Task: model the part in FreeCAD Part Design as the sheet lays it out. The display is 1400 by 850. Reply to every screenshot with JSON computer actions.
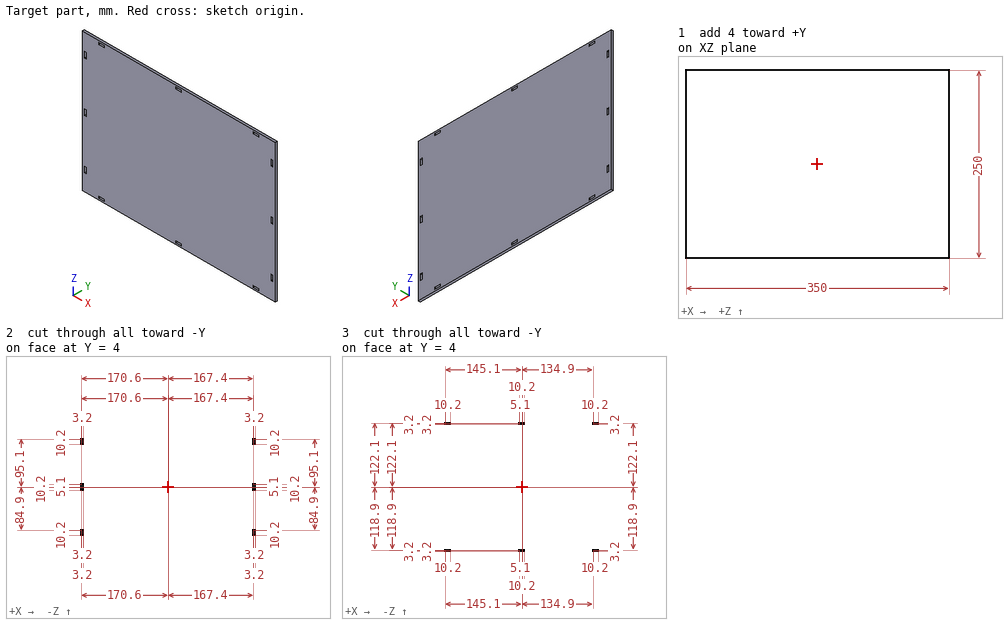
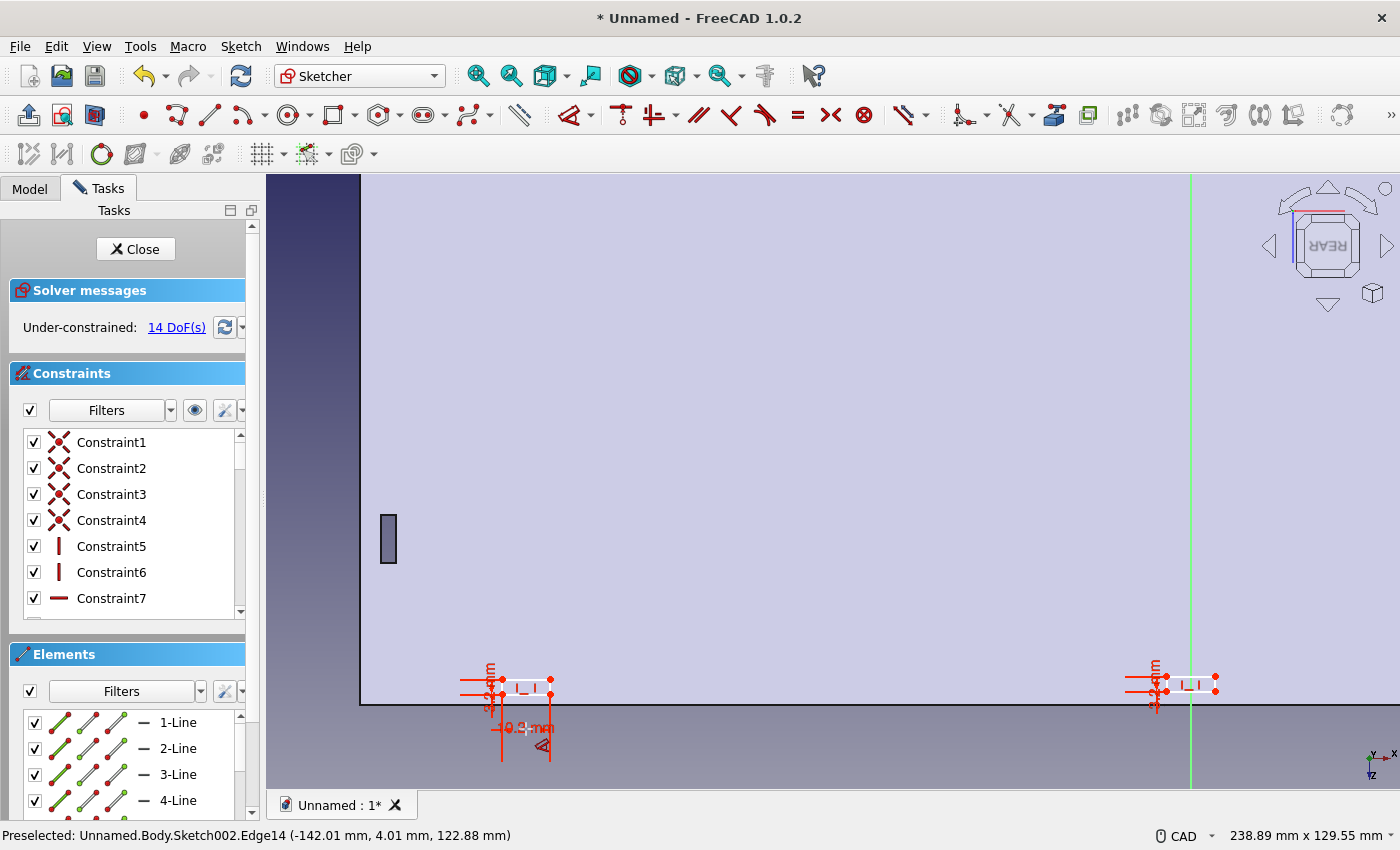
{"action": "scroll", "coordinate": [516, 697], "scroll_direction": "down", "scroll_amount": 5}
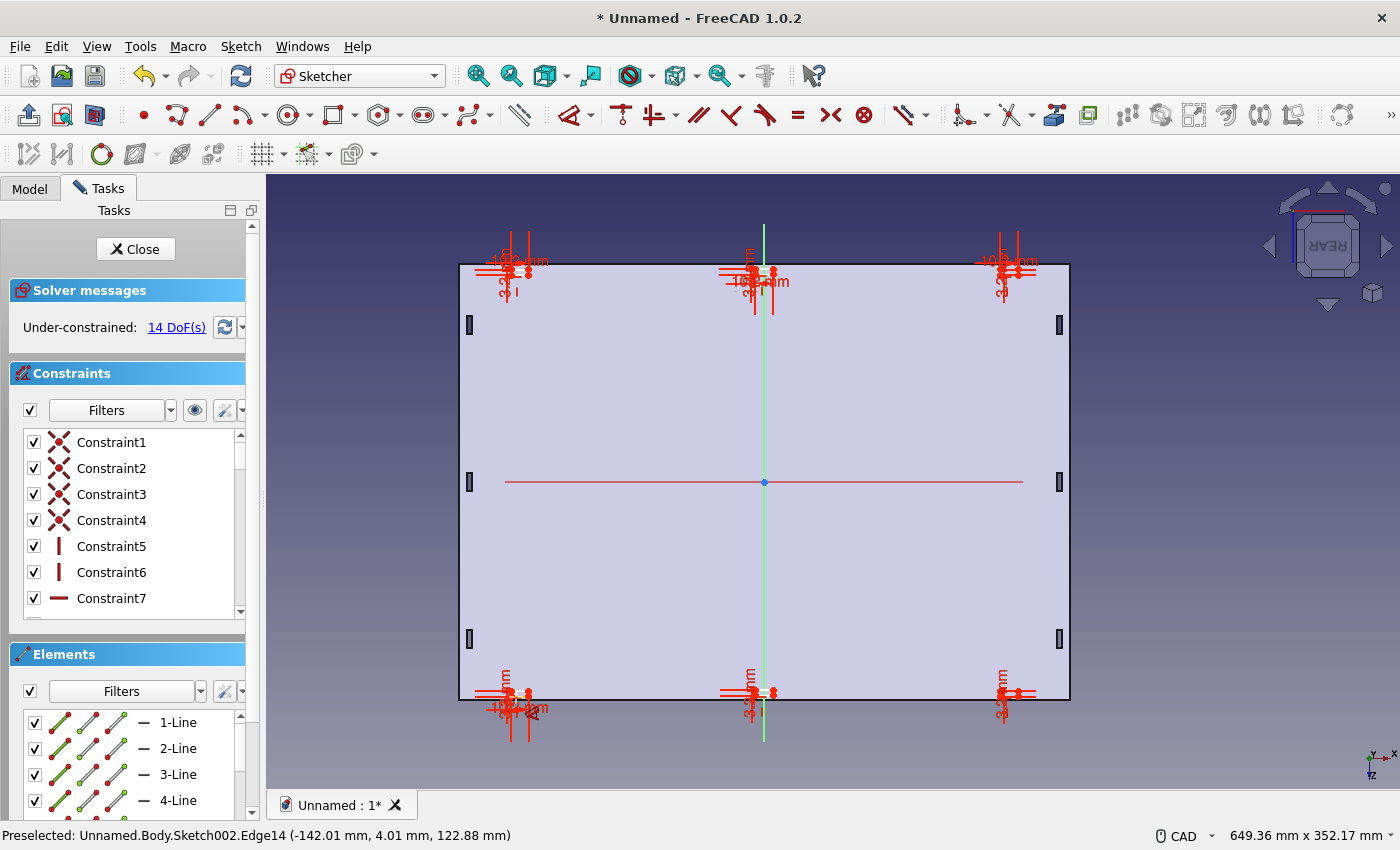
{"action": "scroll", "coordinate": [1006, 697], "scroll_direction": "up", "scroll_amount": 5}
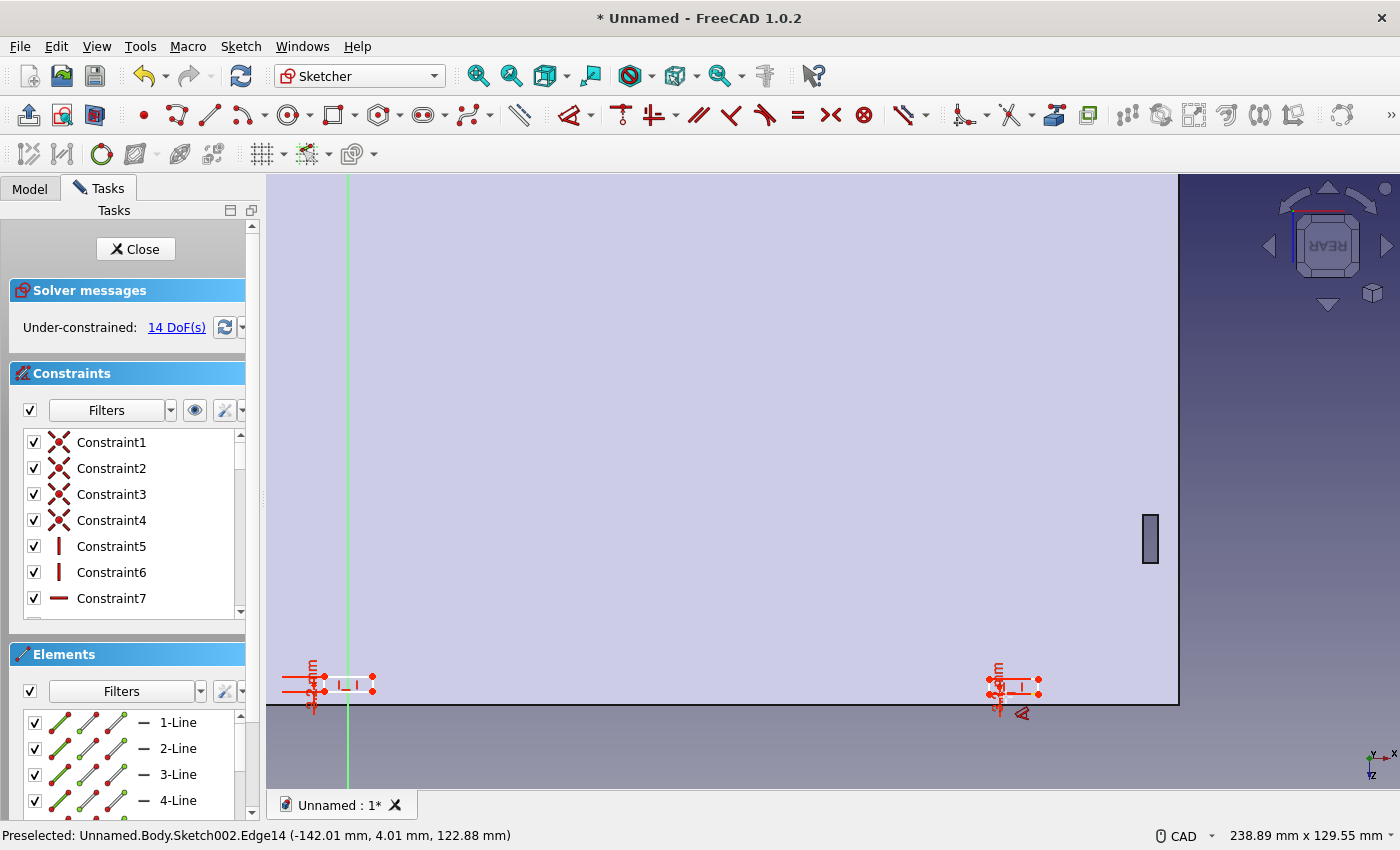
{"action": "left_click", "coordinate": [1004, 694]}
{"action": "left_click", "coordinate": [1014, 728]}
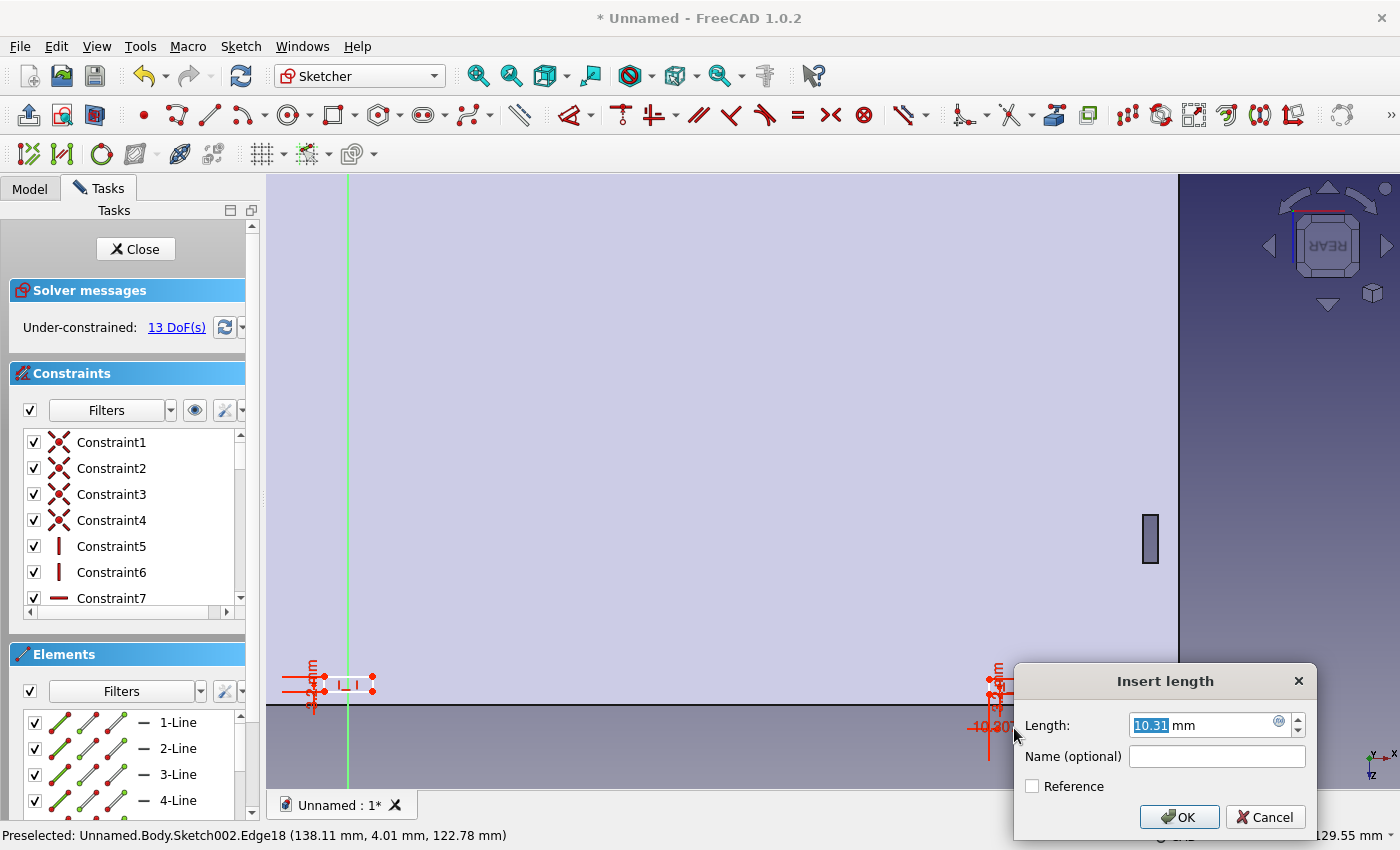
{"action": "type", "text": "10.2"}
{"action": "key", "text": "Return"}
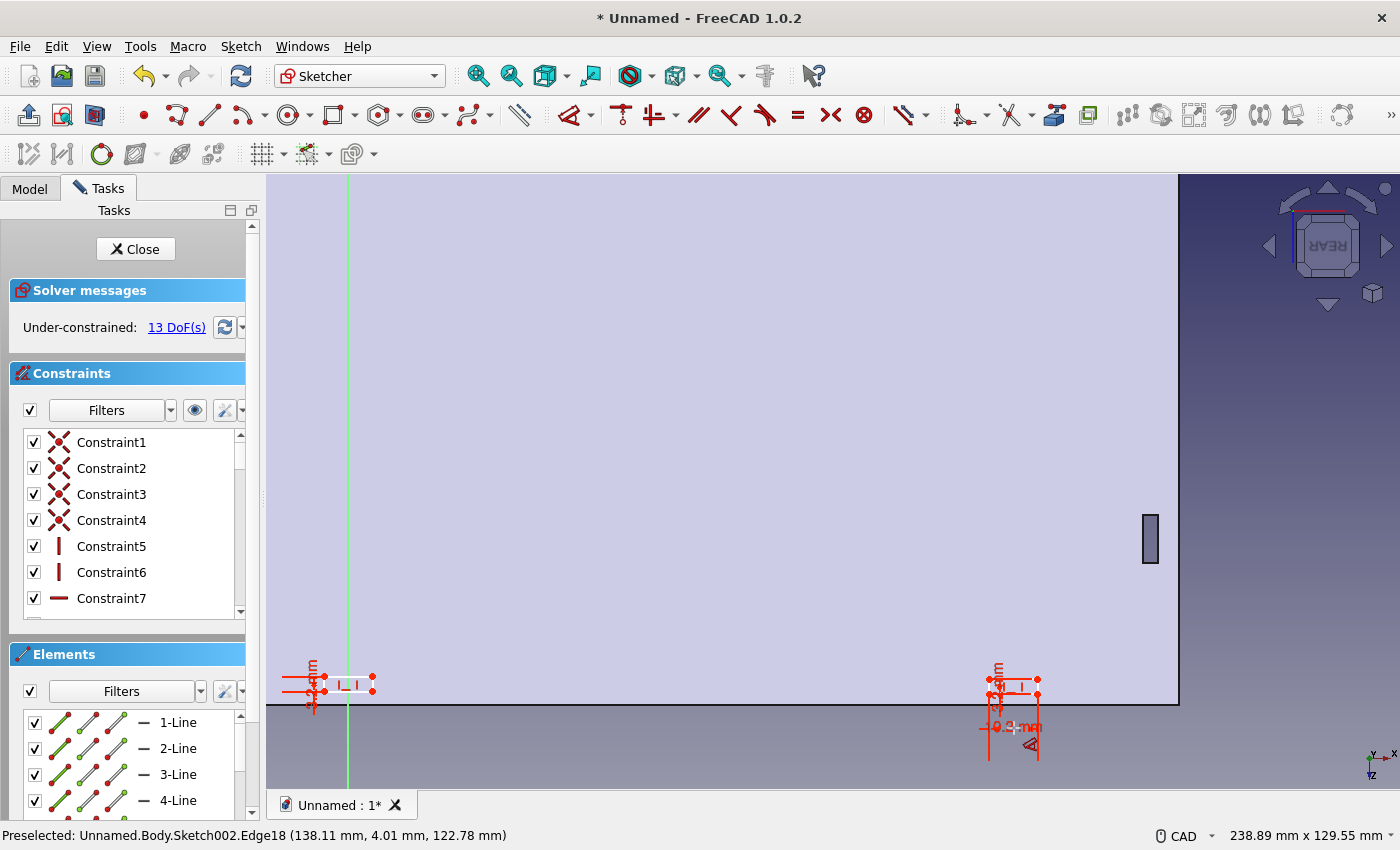
{"action": "scroll", "coordinate": [339, 692], "scroll_direction": "up", "scroll_amount": 2}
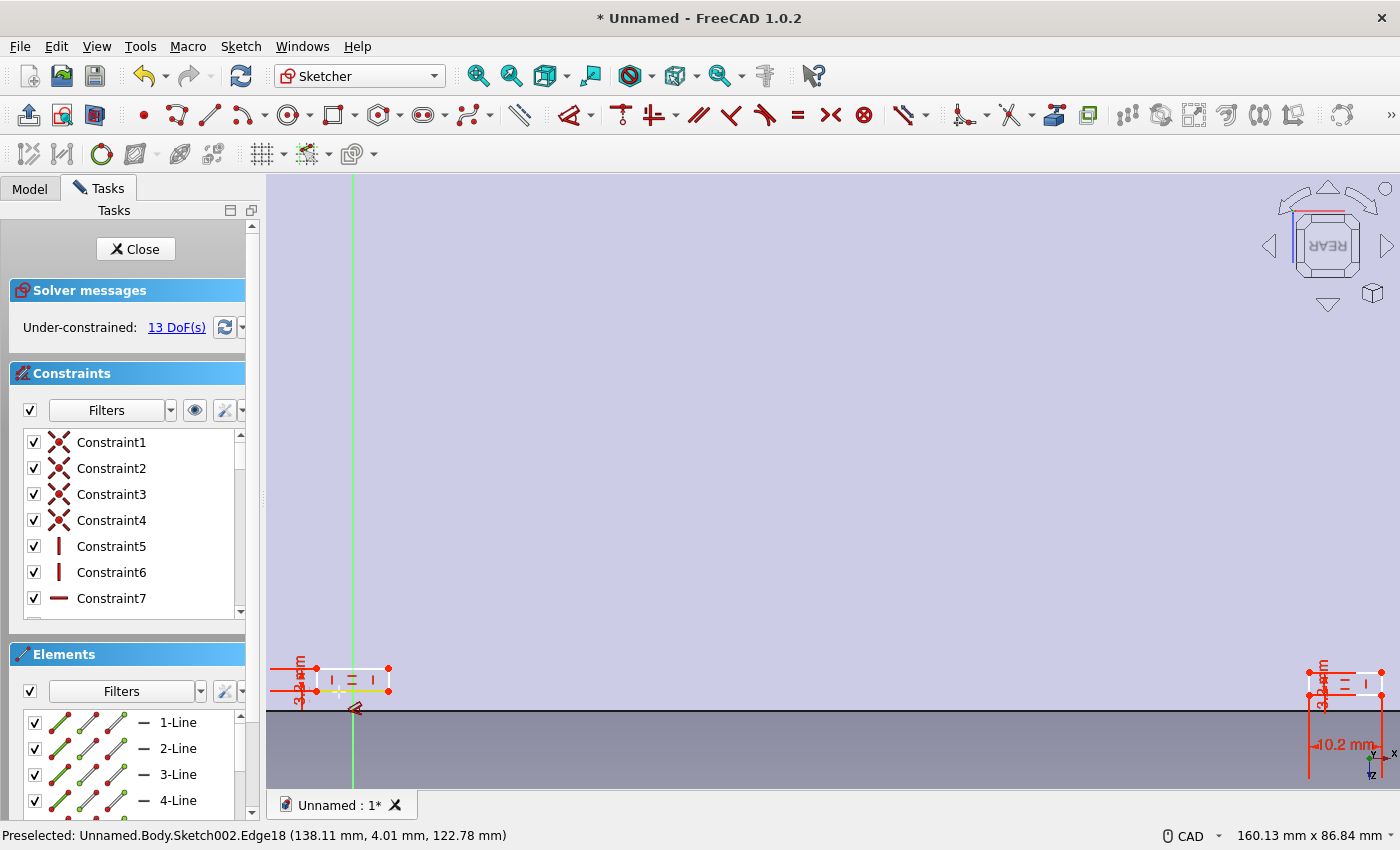
{"action": "left_click", "coordinate": [339, 691]}
{"action": "left_click", "coordinate": [336, 725]}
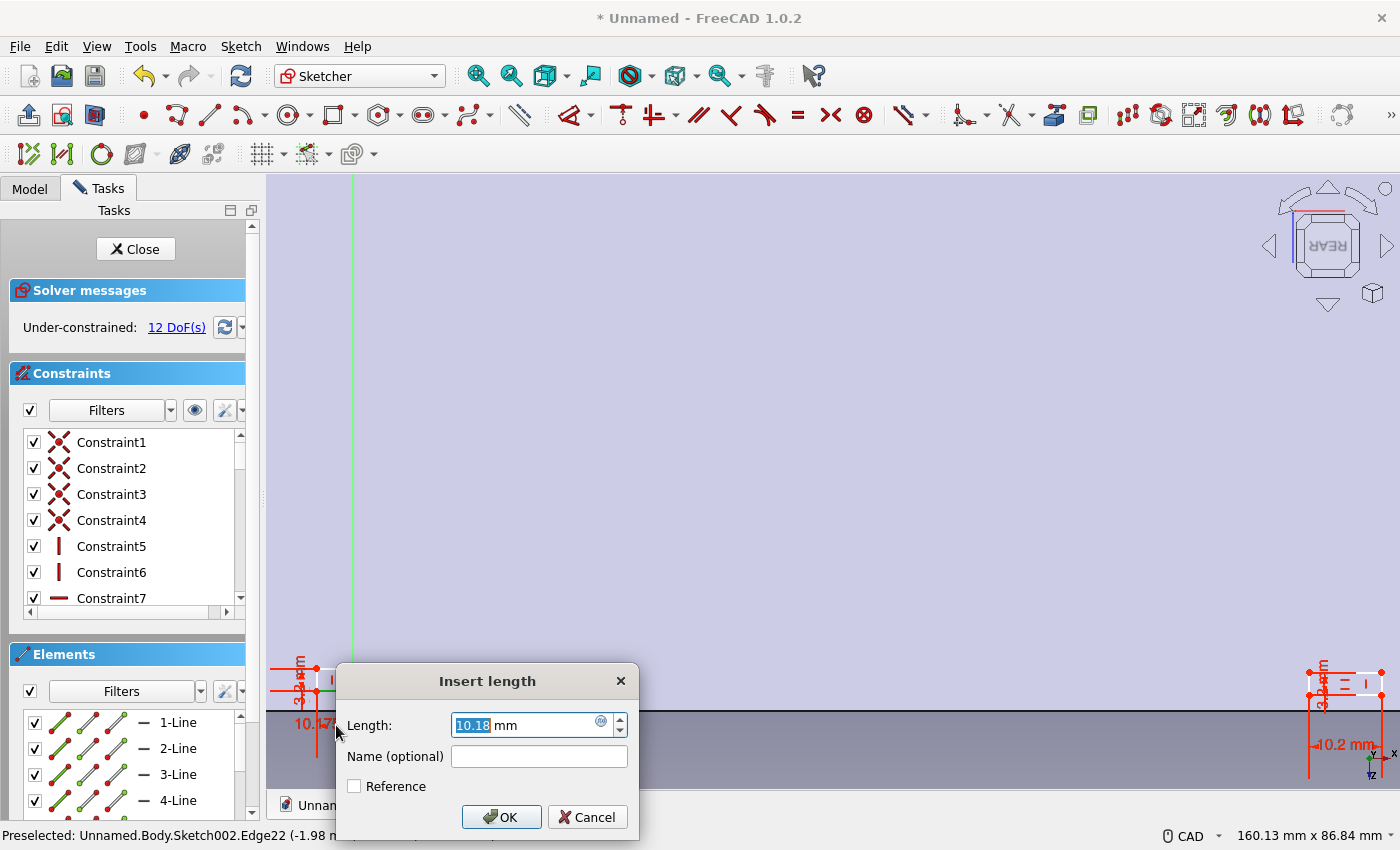
{"action": "type", "text": "10.2"}
{"action": "key", "text": "Return"}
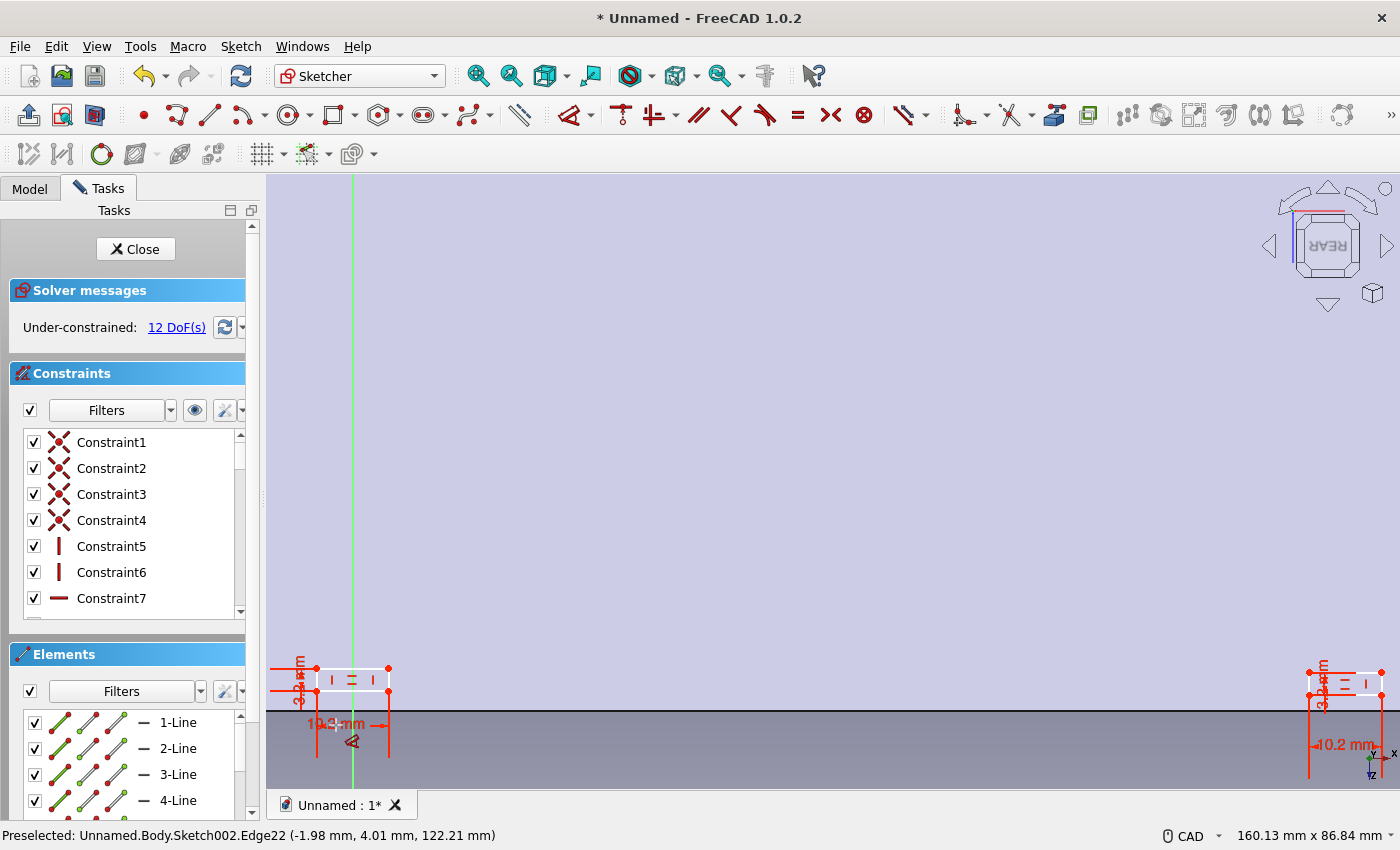
{"action": "scroll", "coordinate": [899, 696], "scroll_direction": "down", "scroll_amount": 7}